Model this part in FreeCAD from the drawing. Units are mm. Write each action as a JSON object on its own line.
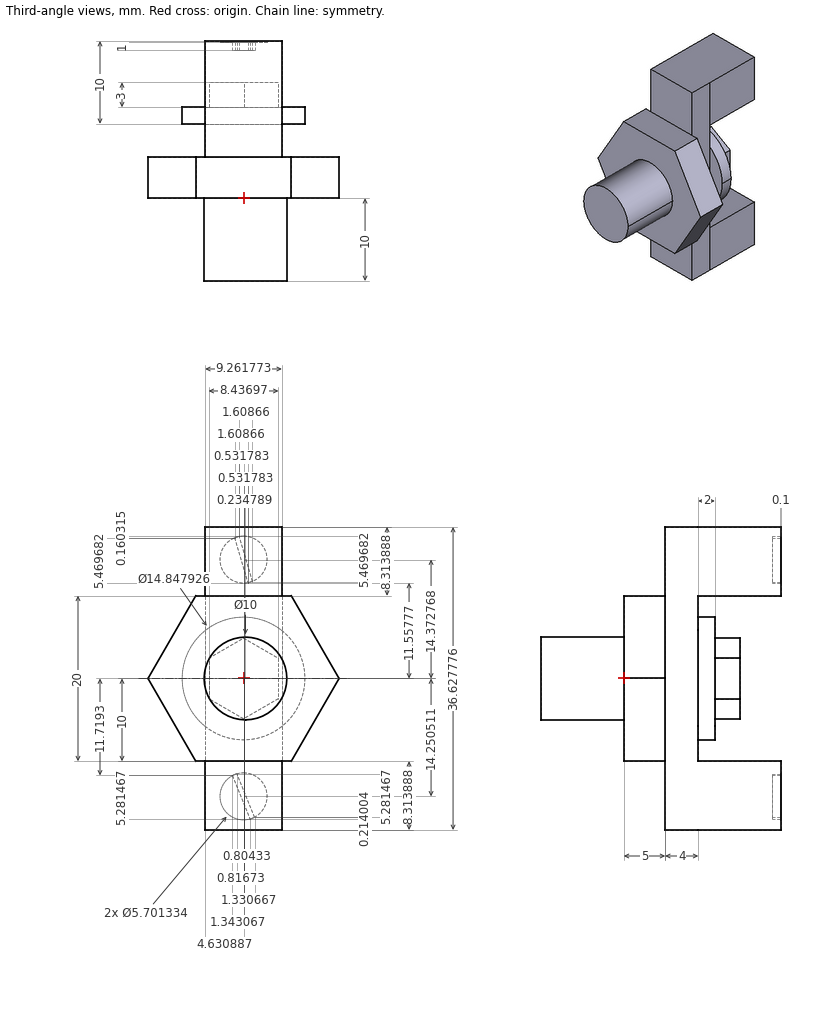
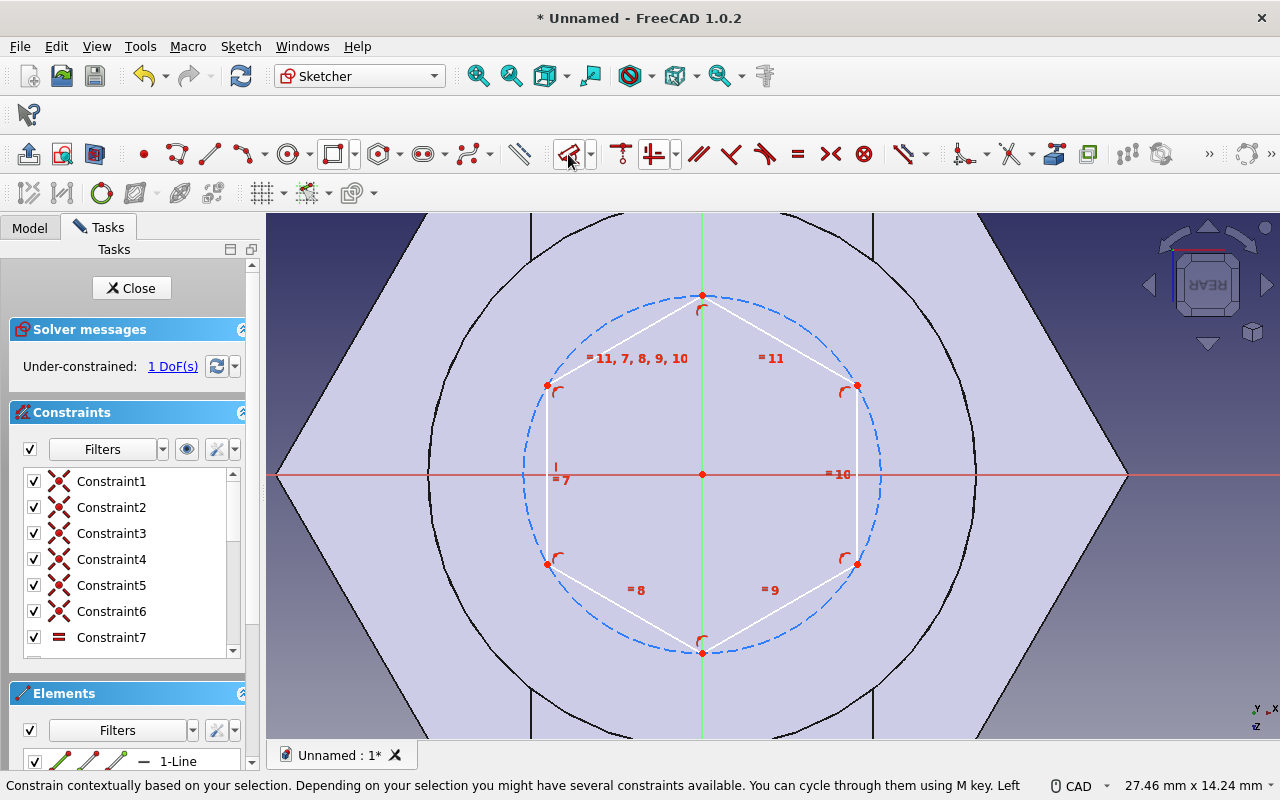
{"action": "left_click", "coordinate": [547, 385]}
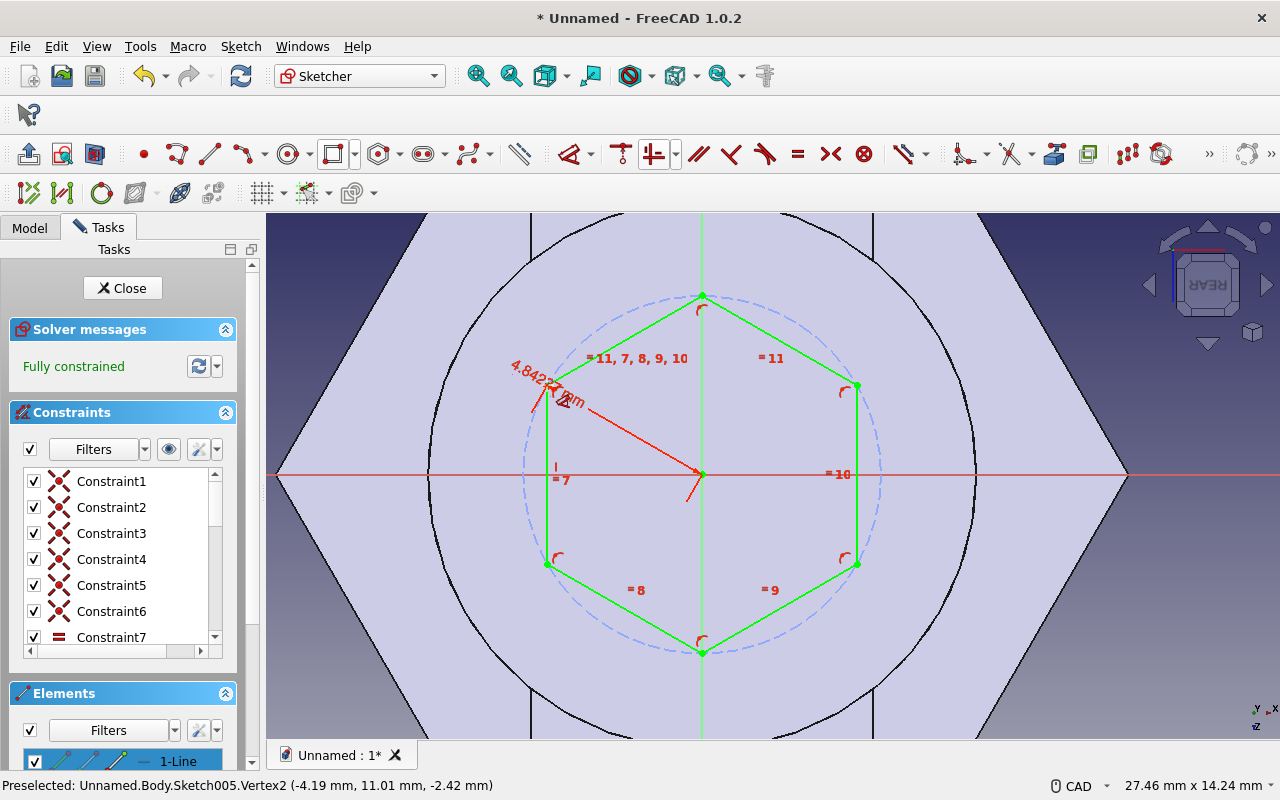
{"action": "left_click", "coordinate": [857, 564]}
{"action": "left_click", "coordinate": [594, 646]}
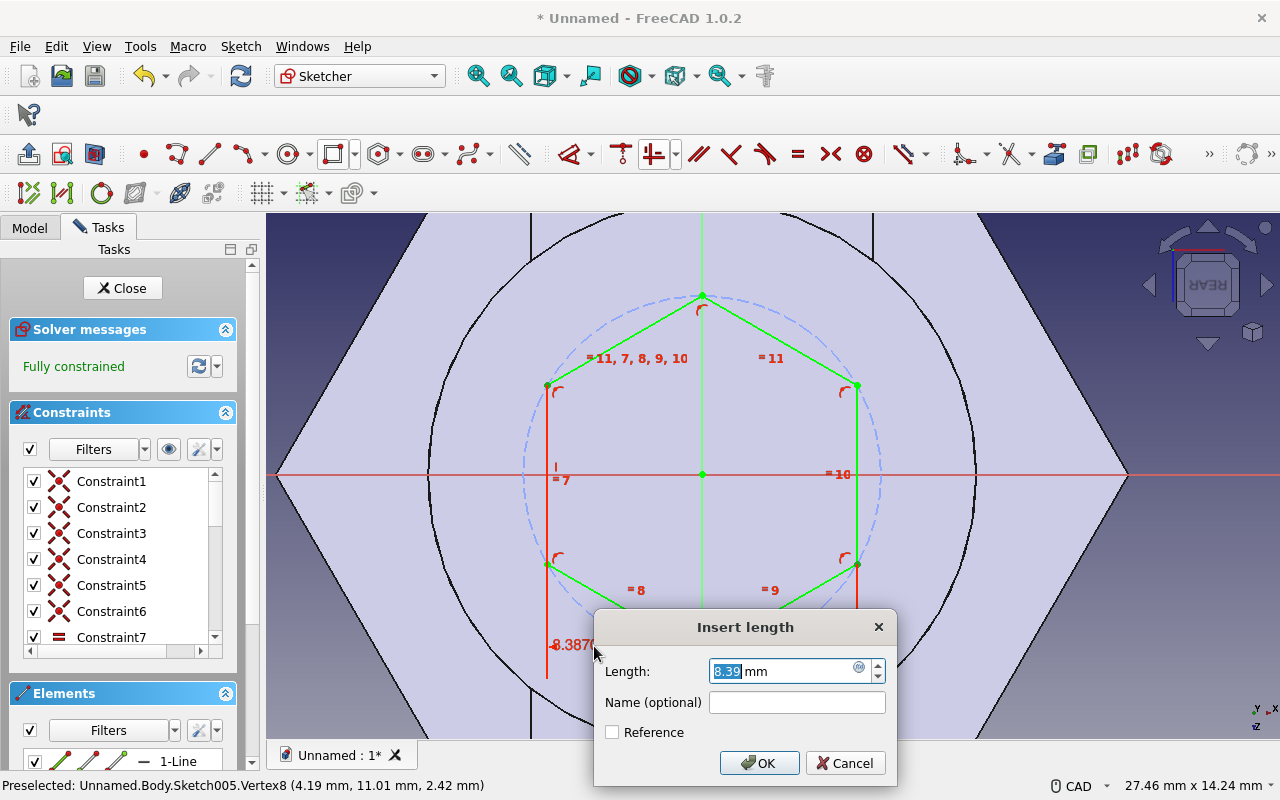
{"action": "type", "text": "8.43697"}
{"action": "key", "text": "Return"}
{"action": "key", "text": "Escape"}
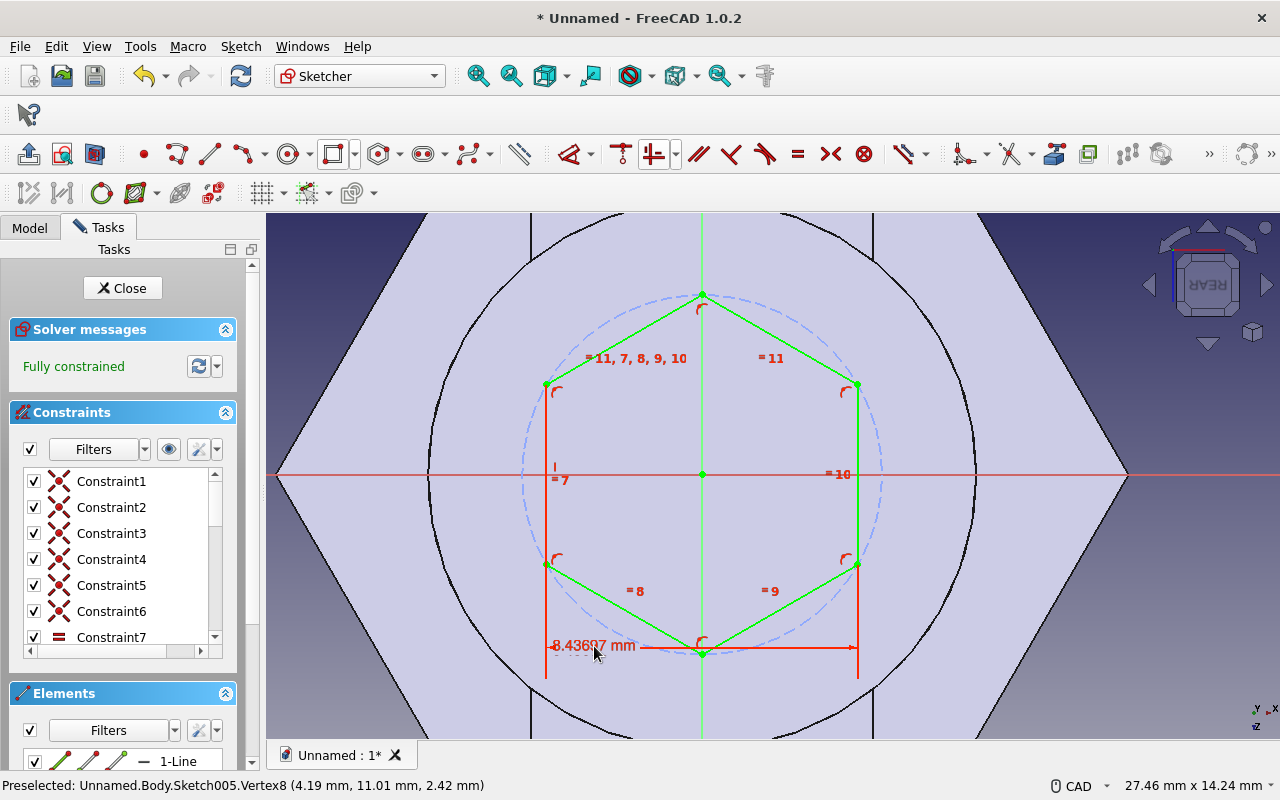
{"action": "left_click", "coordinate": [123, 288]}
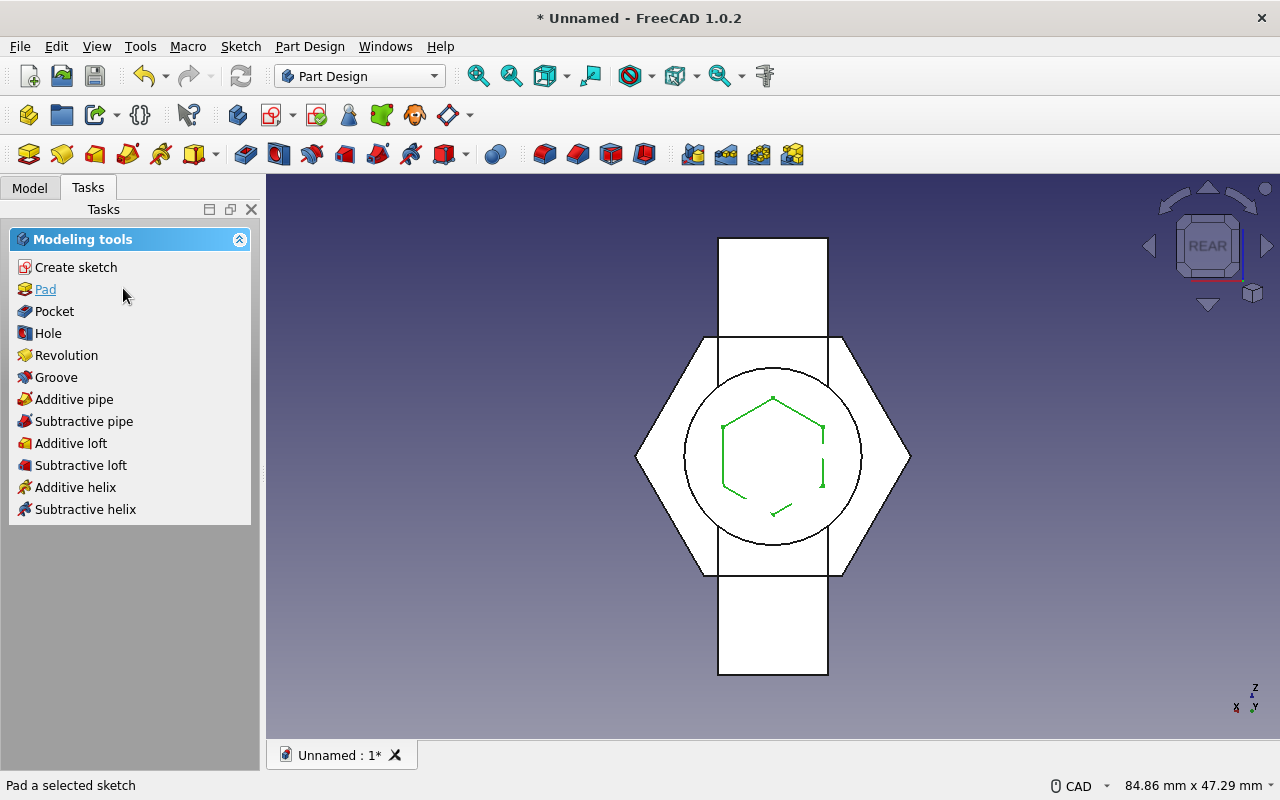
{"action": "left_click", "coordinate": [29, 154]}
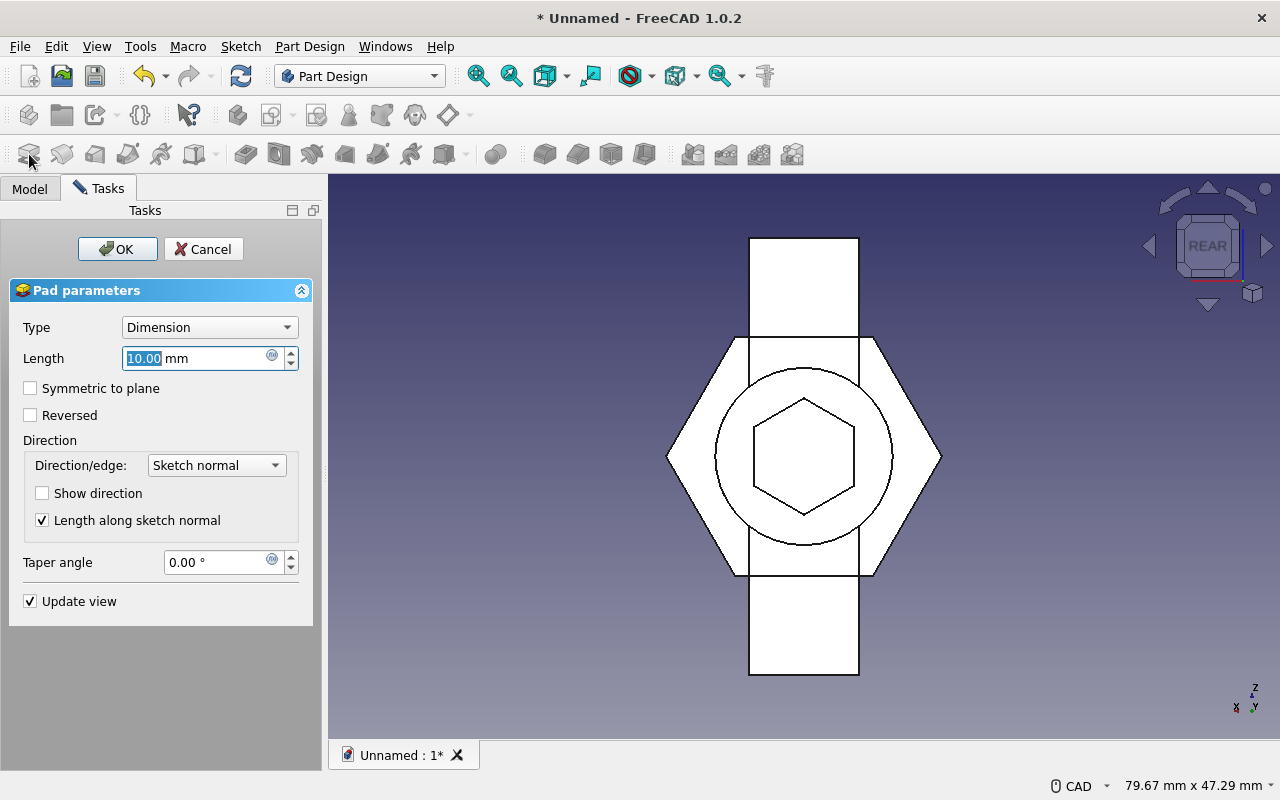
{"action": "type", "text": "3"}
{"action": "key", "text": "Tab"}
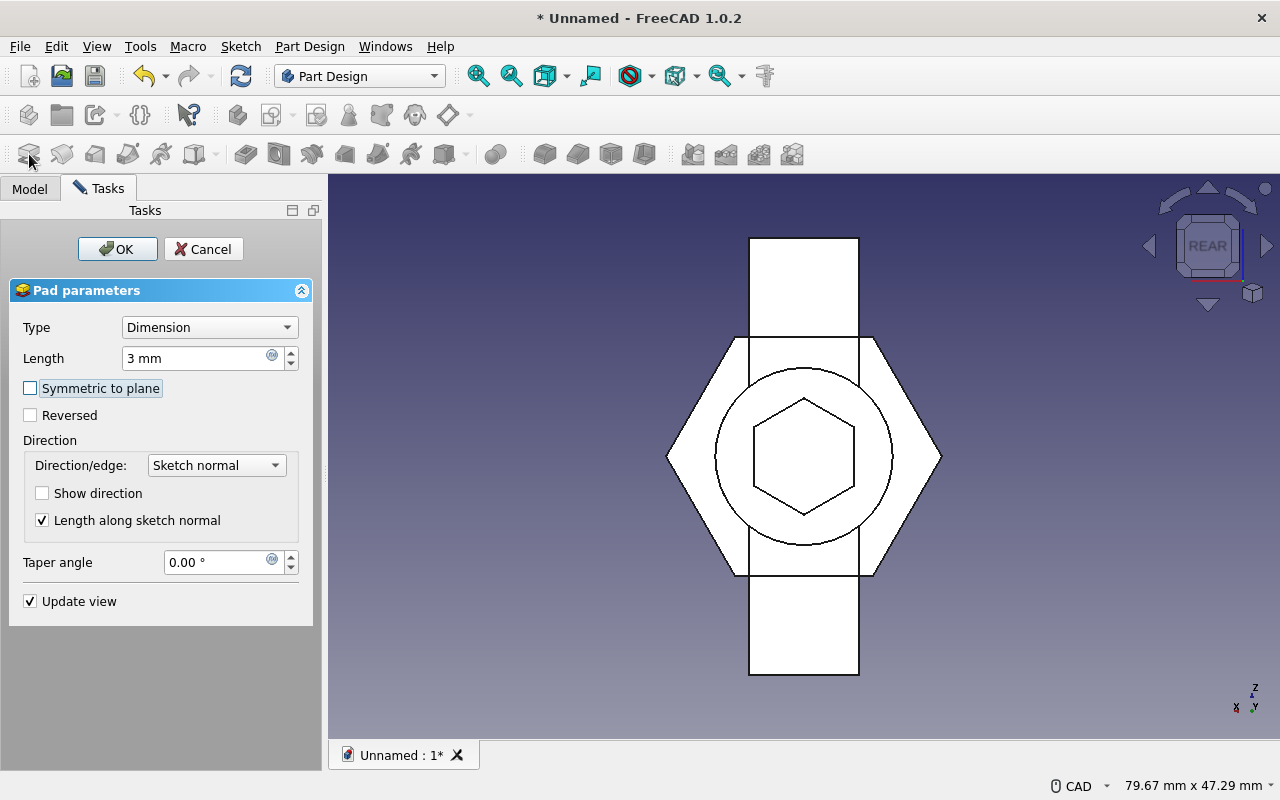
{"action": "left_click", "coordinate": [118, 249]}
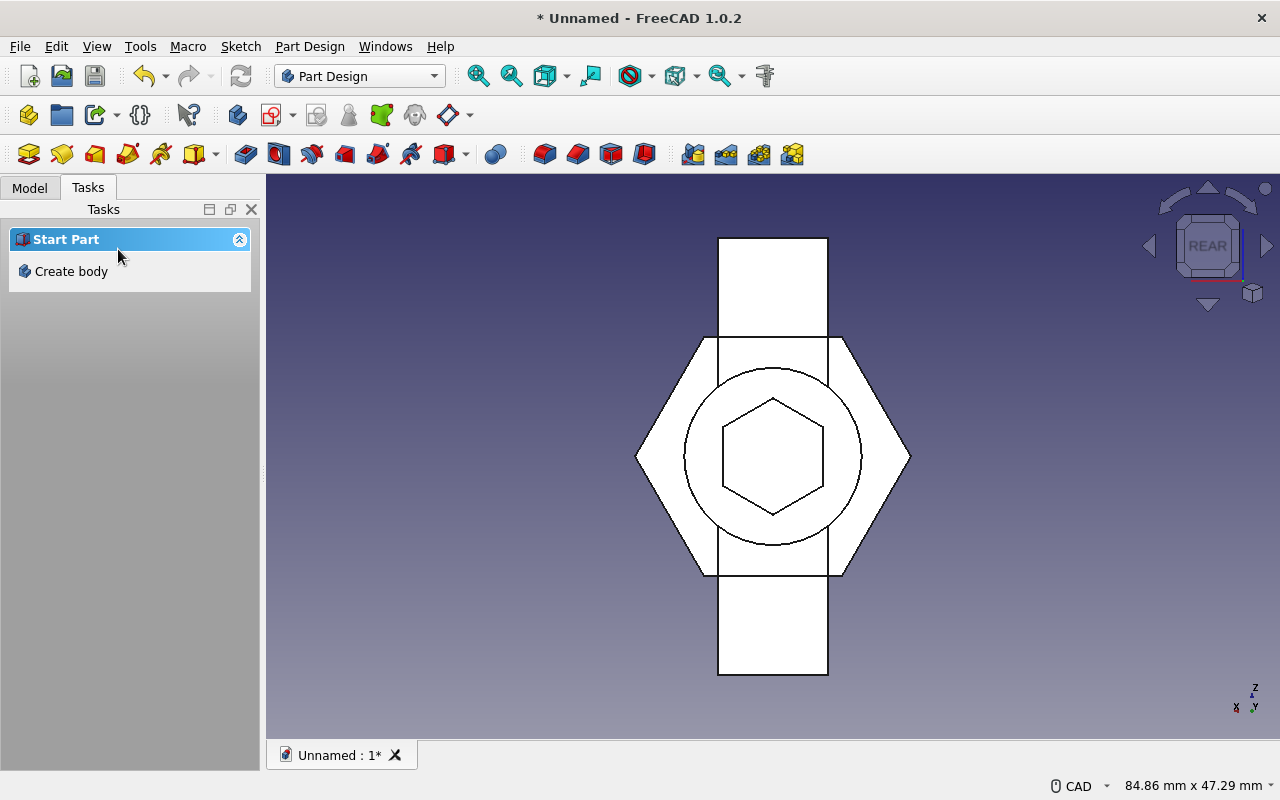
{"action": "left_click", "coordinate": [773, 286]}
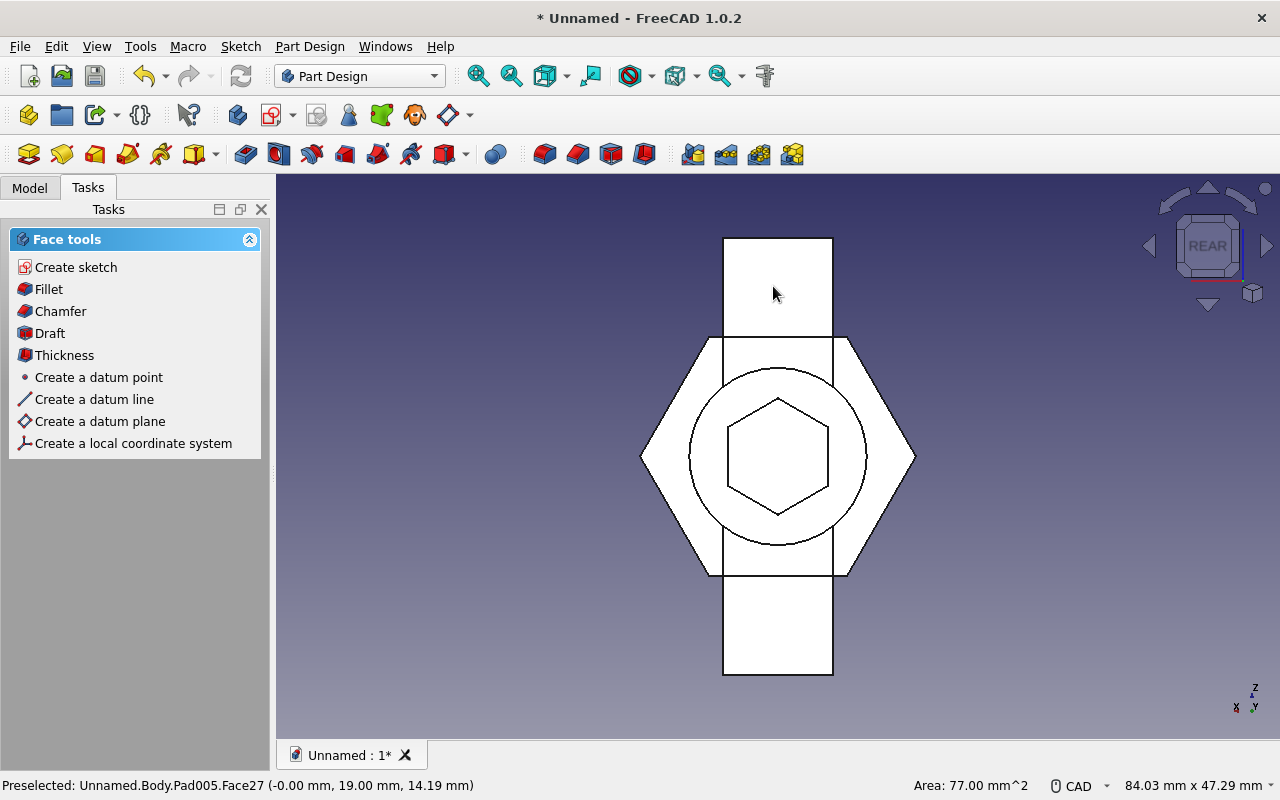
{"action": "left_click", "coordinate": [270, 116]}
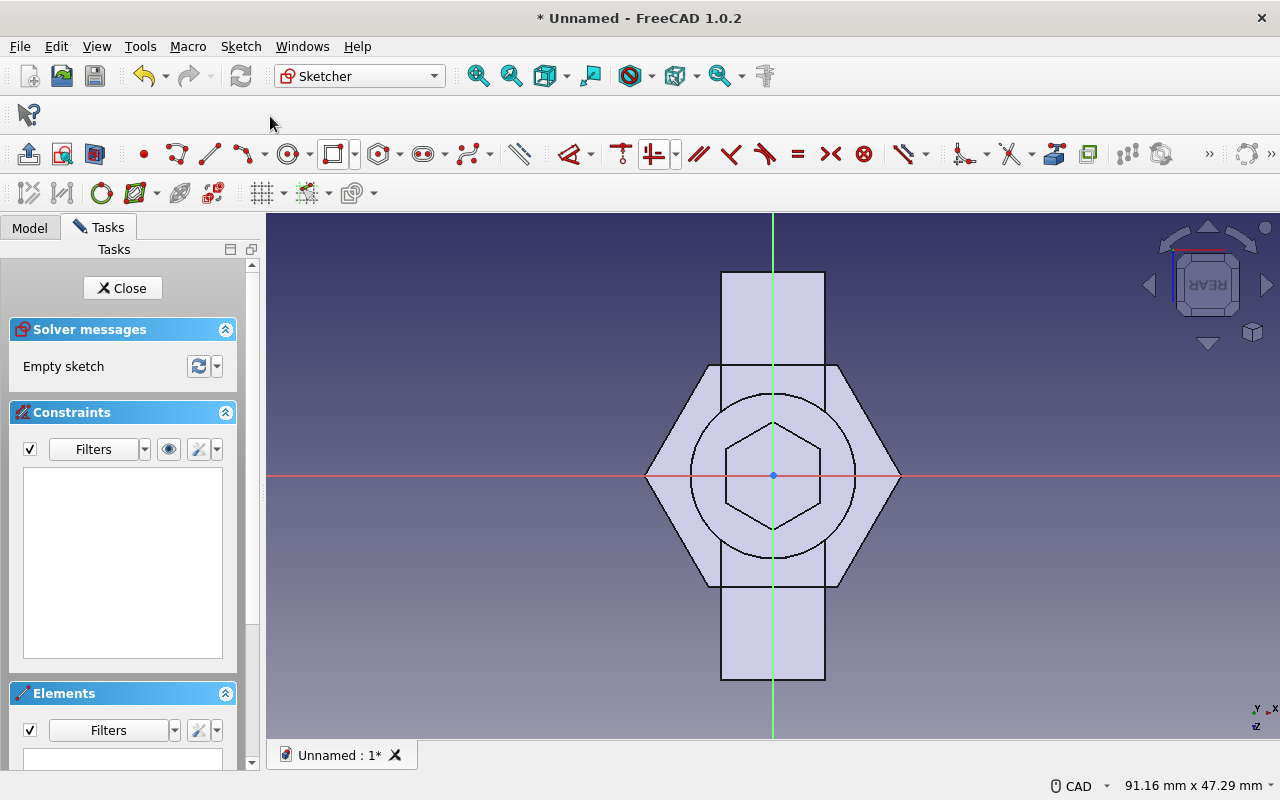
{"action": "left_click", "coordinate": [288, 154]}